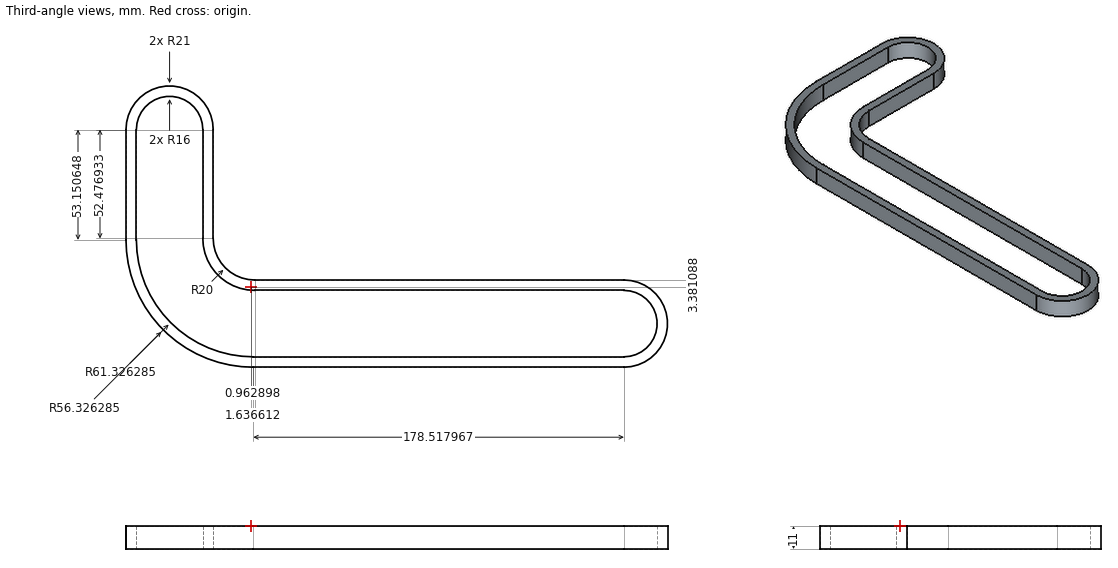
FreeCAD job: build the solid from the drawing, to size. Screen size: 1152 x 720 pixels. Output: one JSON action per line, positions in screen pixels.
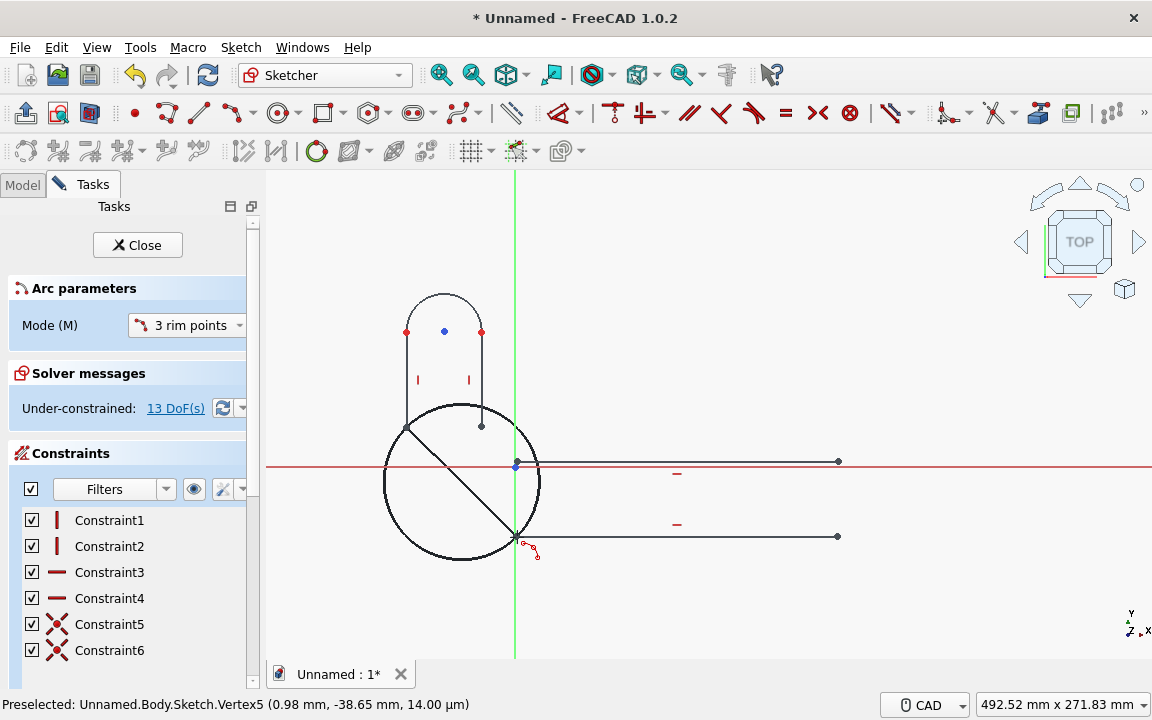
{"action": "left_click", "coordinate": [439, 505]}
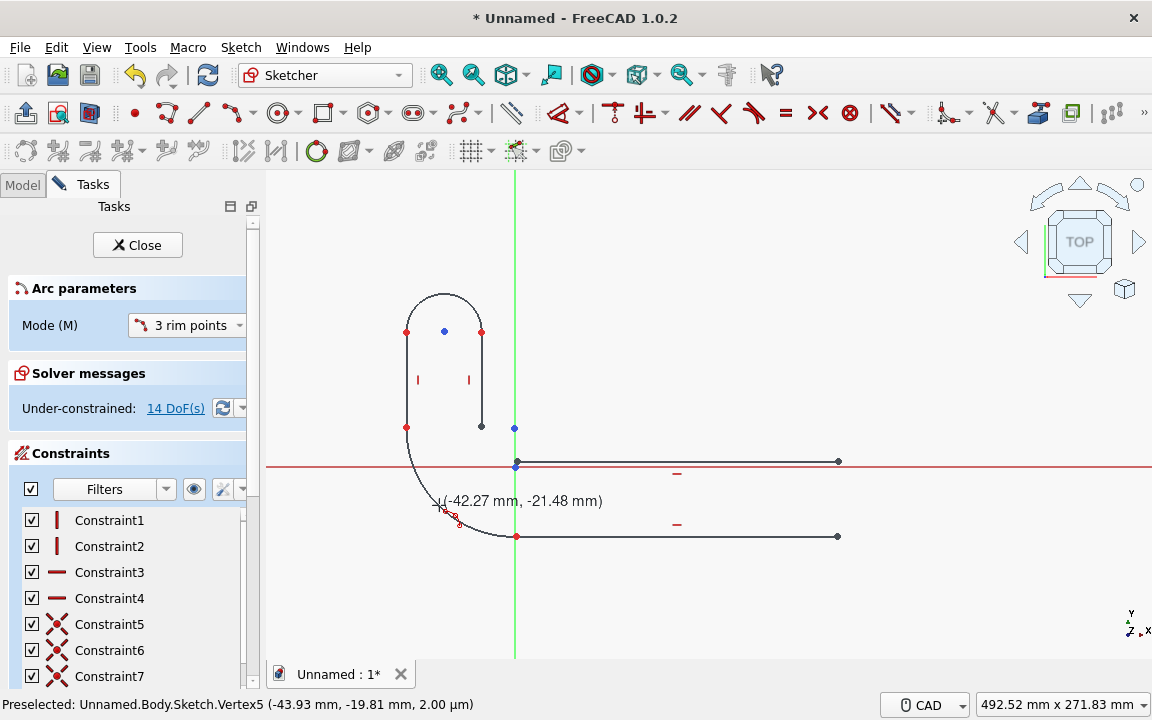
{"action": "left_click", "coordinate": [838, 537]}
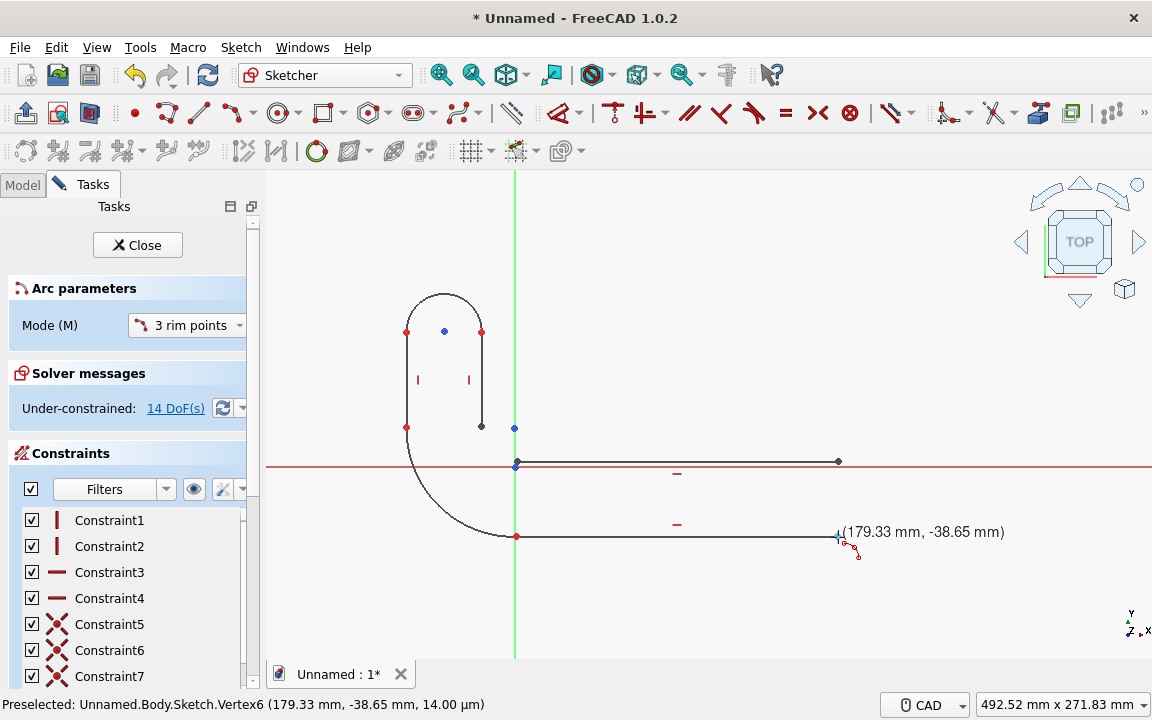
{"action": "scroll", "coordinate": [838, 461], "scroll_direction": "up", "scroll_amount": 5}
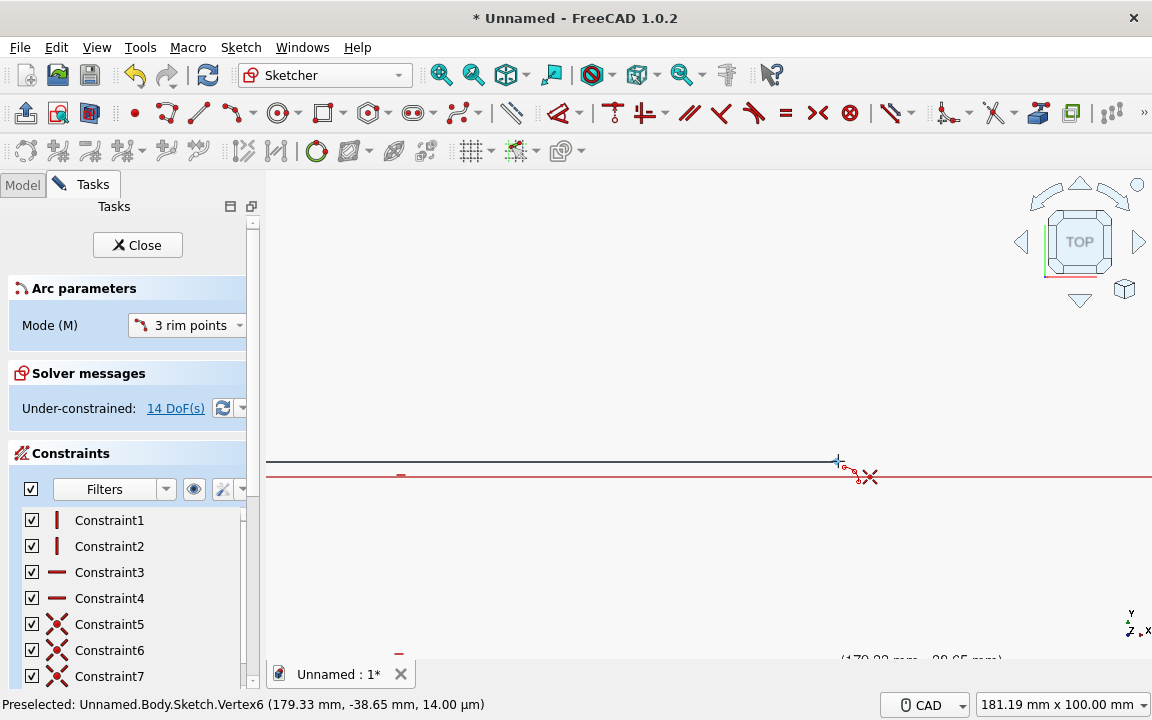
{"action": "left_click", "coordinate": [837, 462]}
{"action": "left_click", "coordinate": [939, 563]}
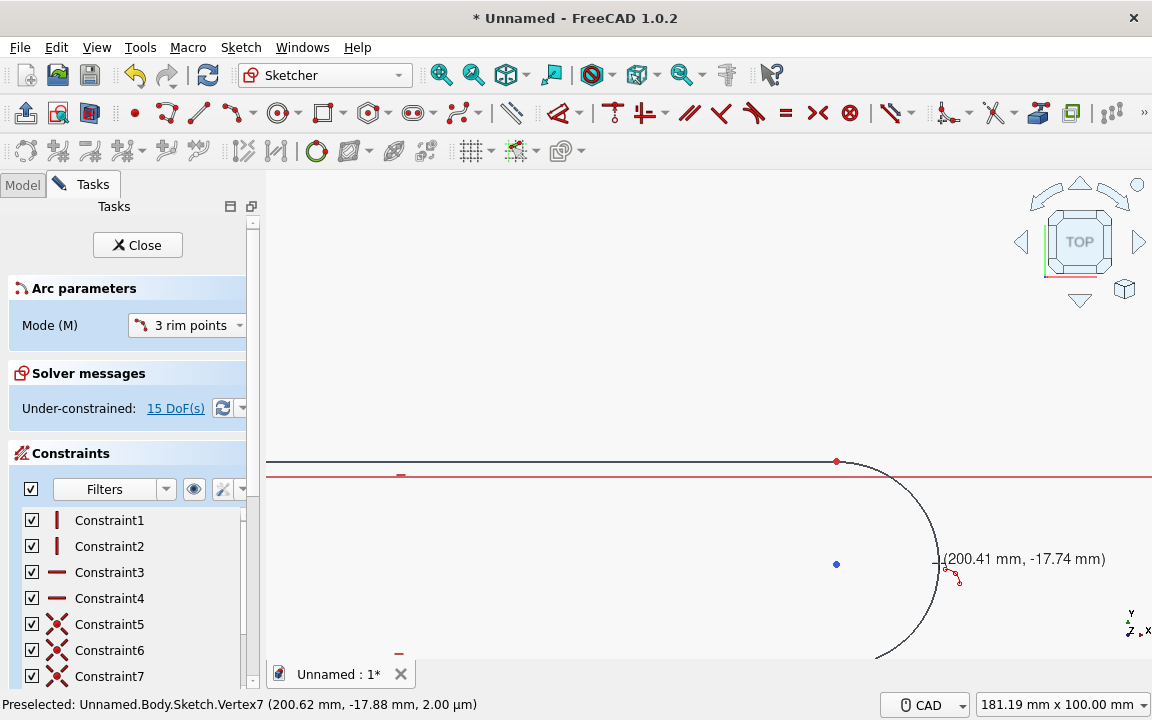
{"action": "scroll", "coordinate": [838, 461], "scroll_direction": "down", "scroll_amount": 5}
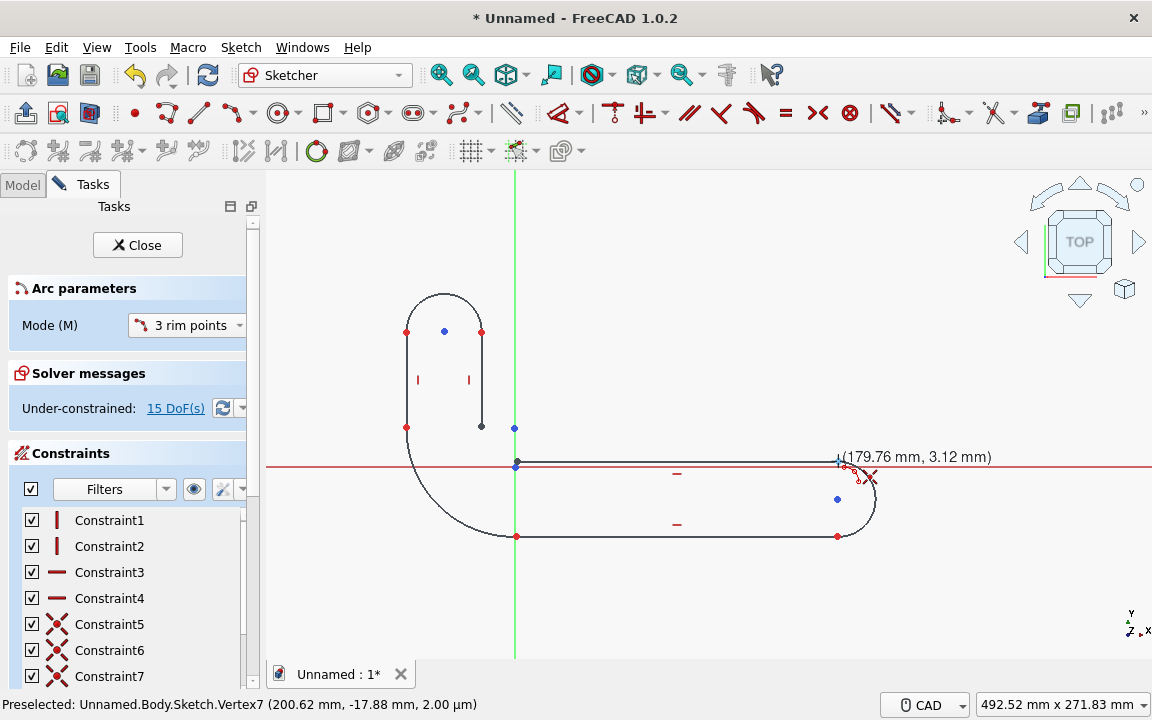
{"action": "scroll", "coordinate": [518, 461], "scroll_direction": "up", "scroll_amount": 9}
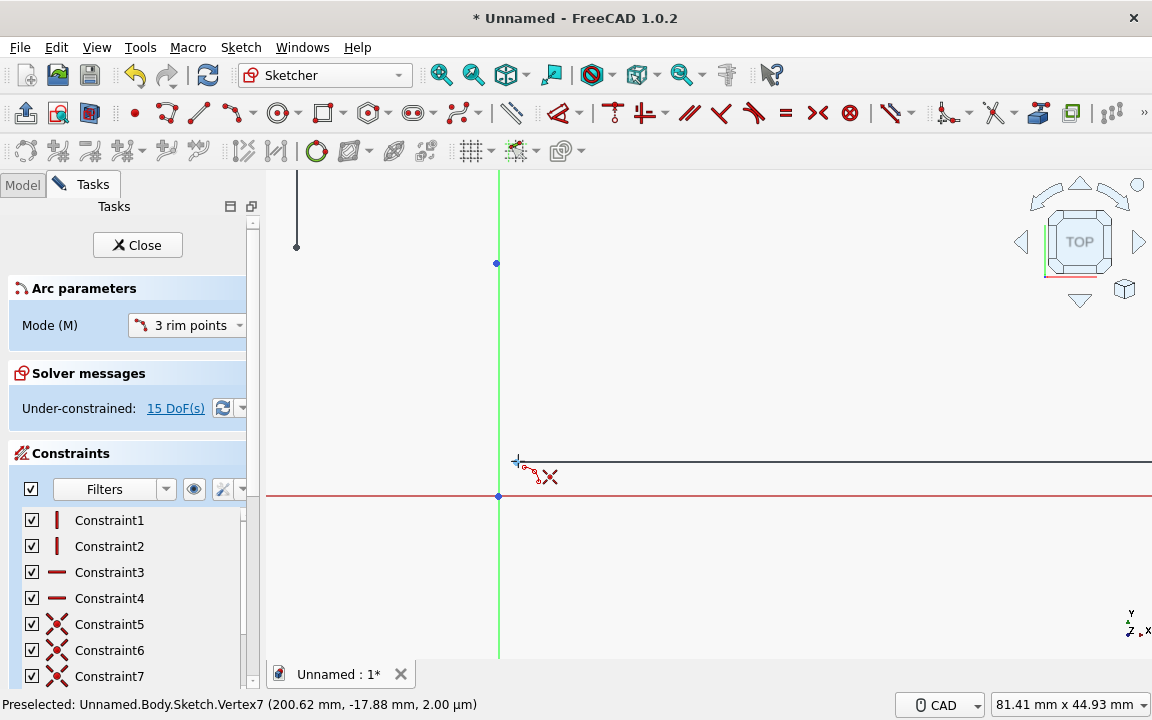
{"action": "left_click", "coordinate": [516, 462]}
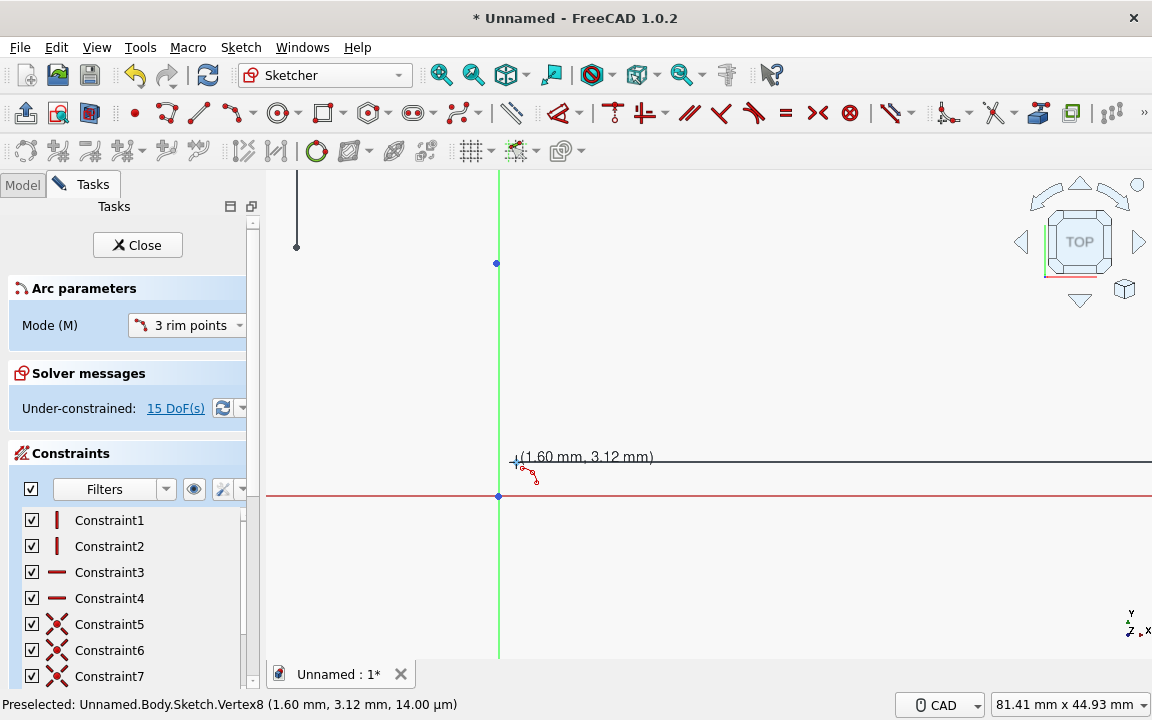
{"action": "scroll", "coordinate": [518, 461], "scroll_direction": "down", "scroll_amount": 9}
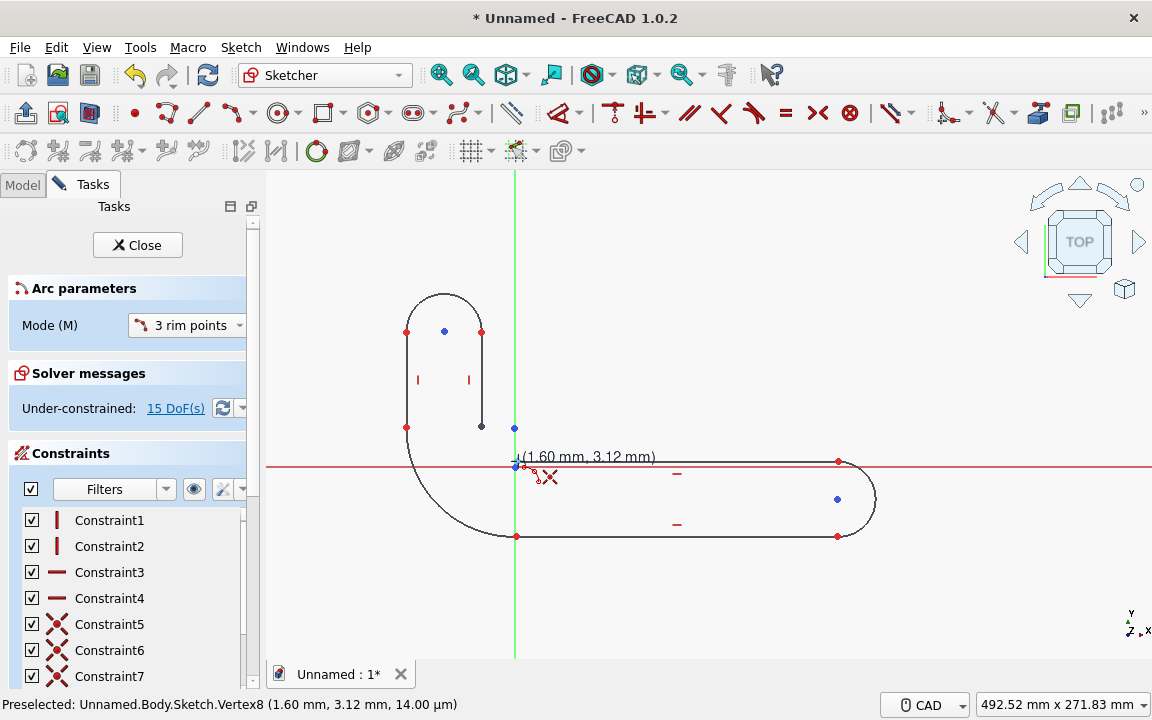
{"action": "left_click", "coordinate": [482, 426]}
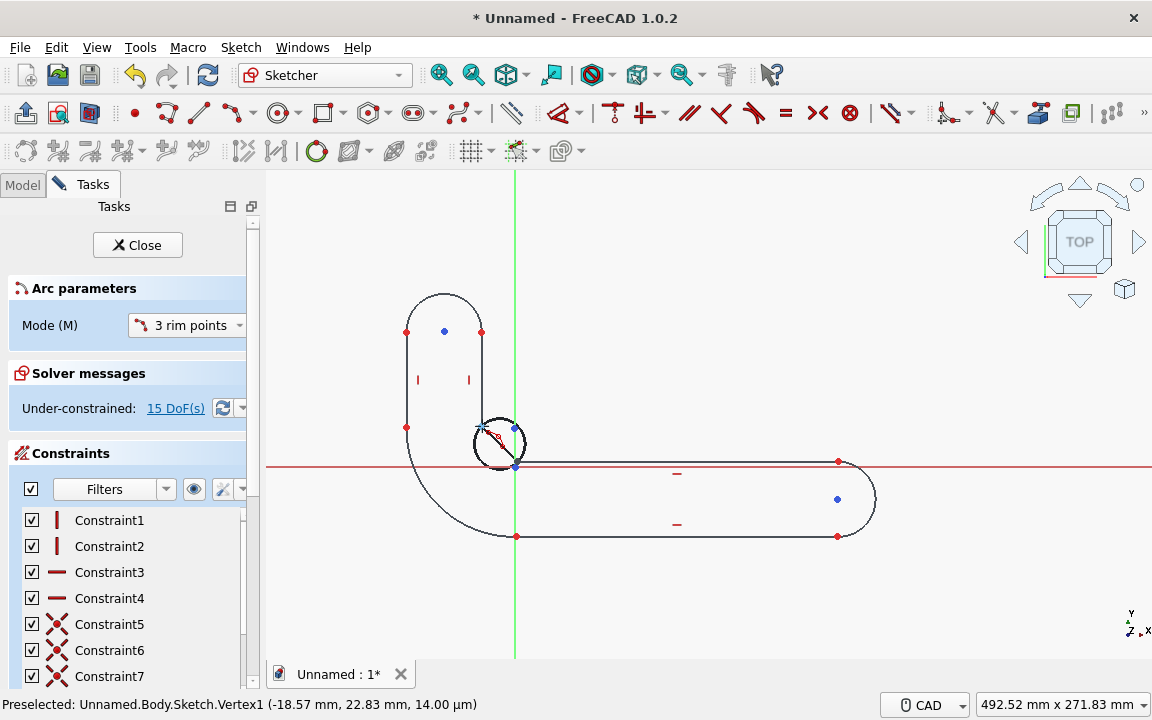
{"action": "scroll", "coordinate": [493, 451], "scroll_direction": "up", "scroll_amount": 3}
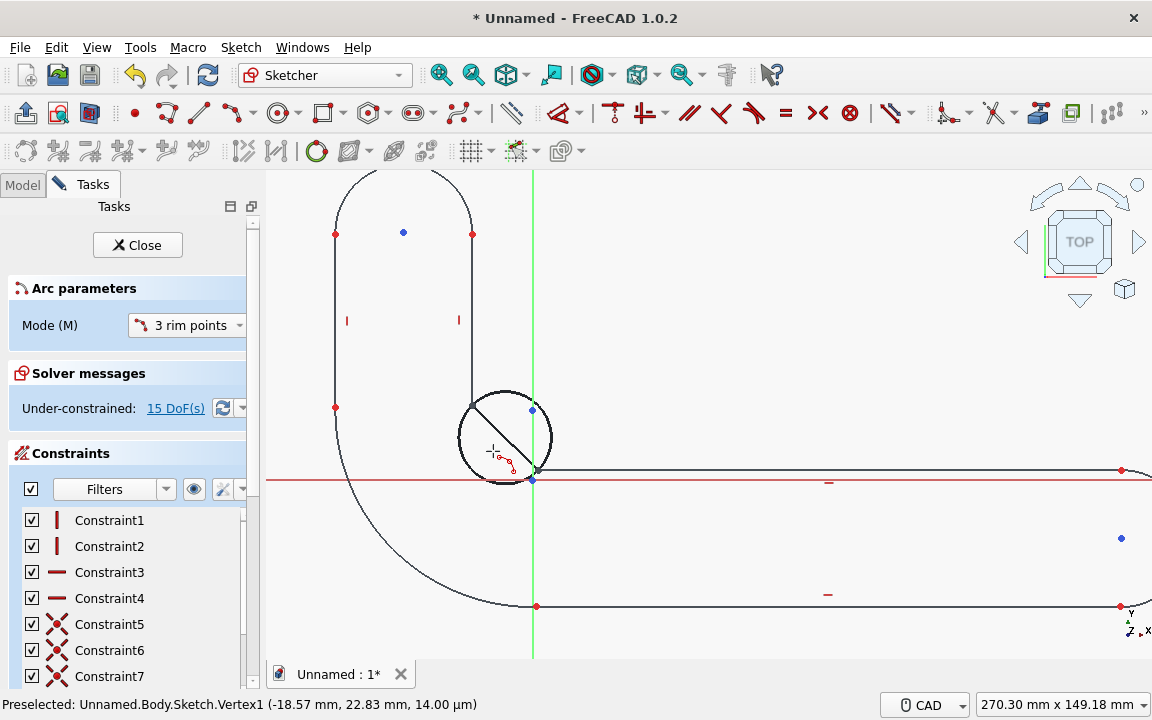
{"action": "left_click", "coordinate": [492, 450]}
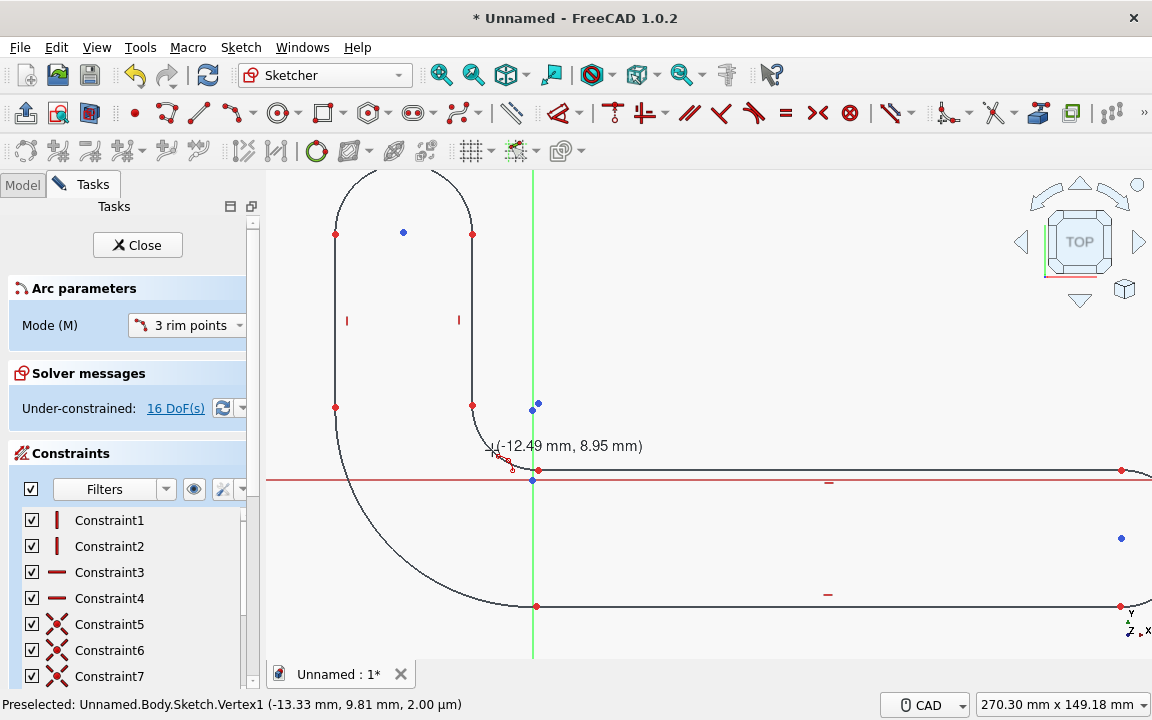
{"action": "left_click", "coordinate": [200, 114]}